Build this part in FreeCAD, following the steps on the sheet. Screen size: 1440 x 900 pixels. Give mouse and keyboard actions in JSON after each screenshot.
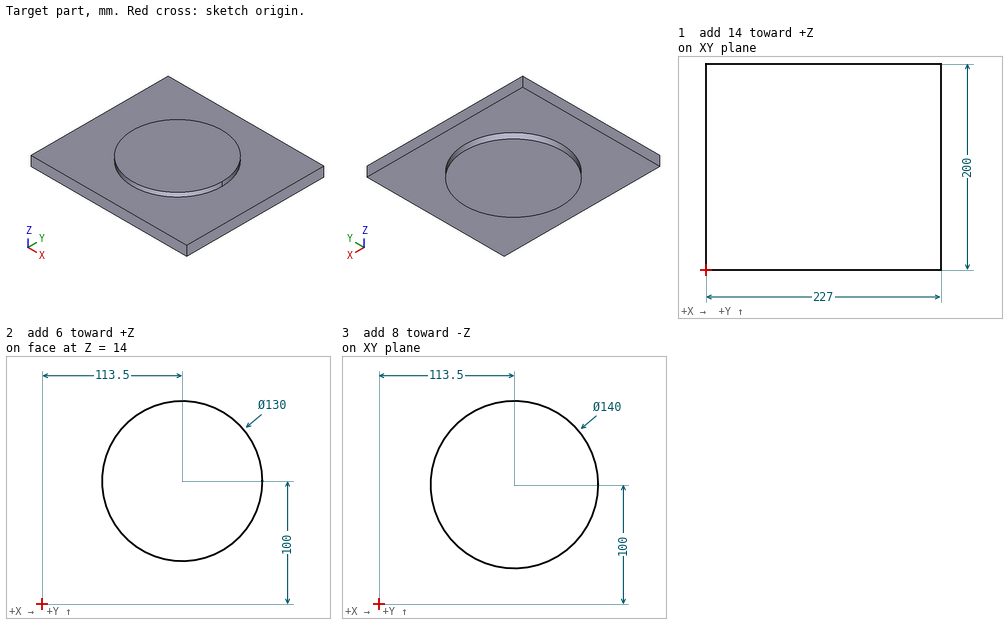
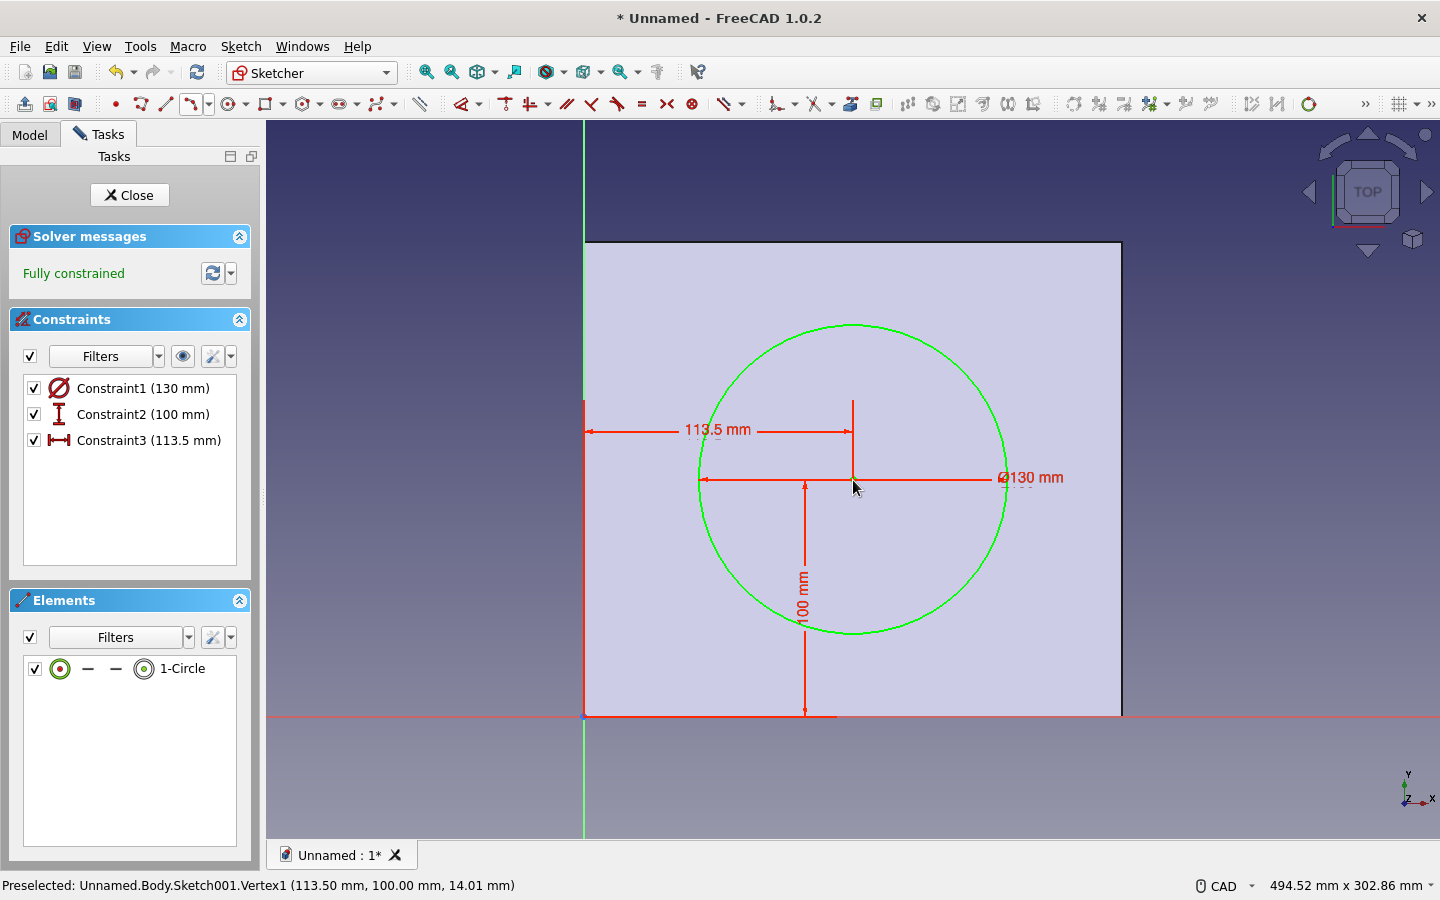
{"action": "left_click", "coordinate": [130, 195]}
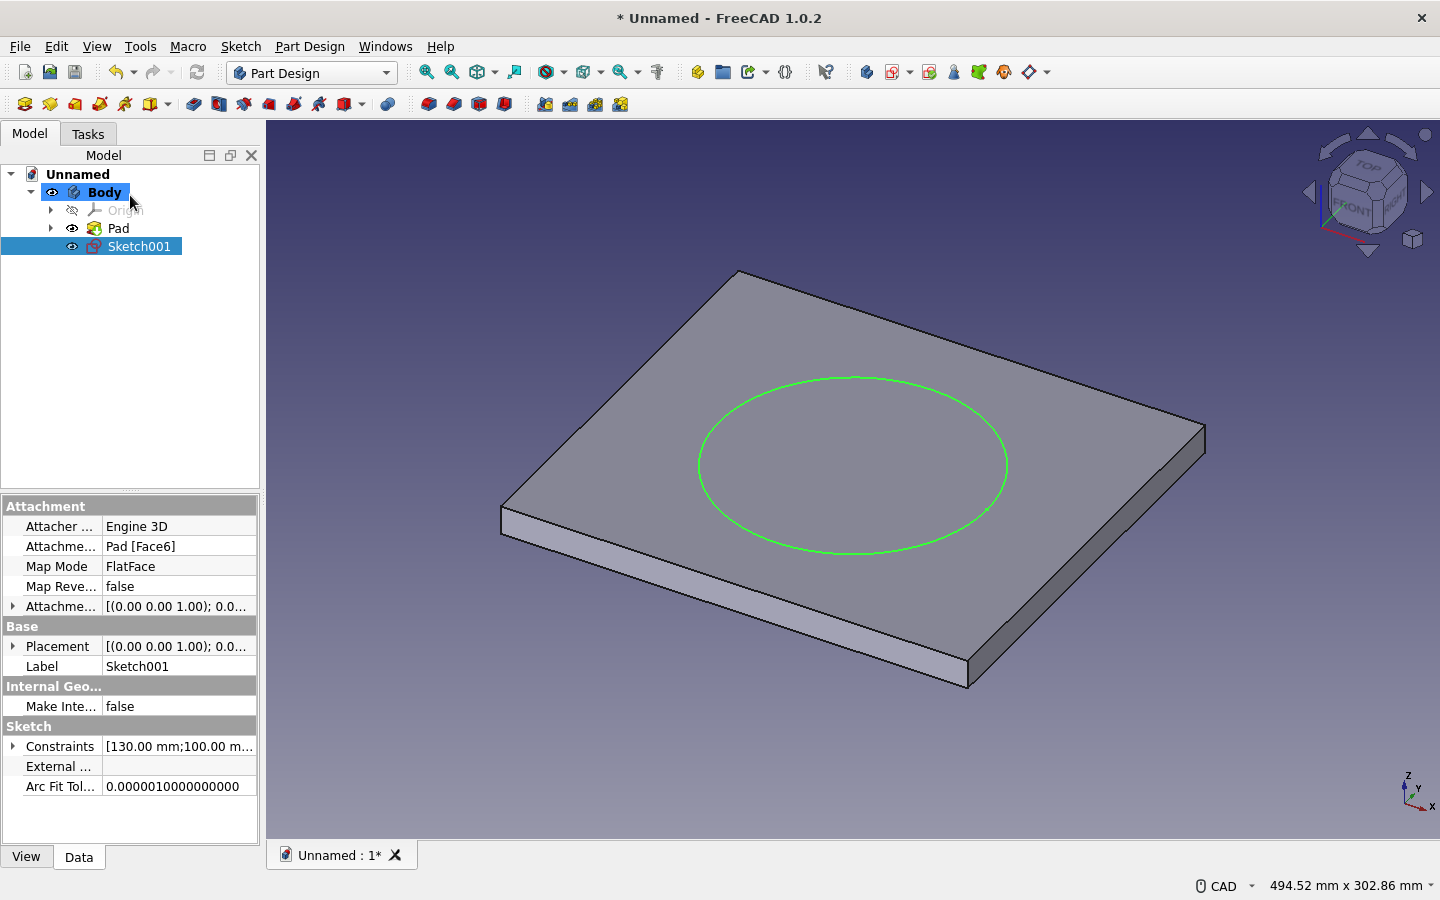
{"action": "left_click", "coordinate": [25, 104]}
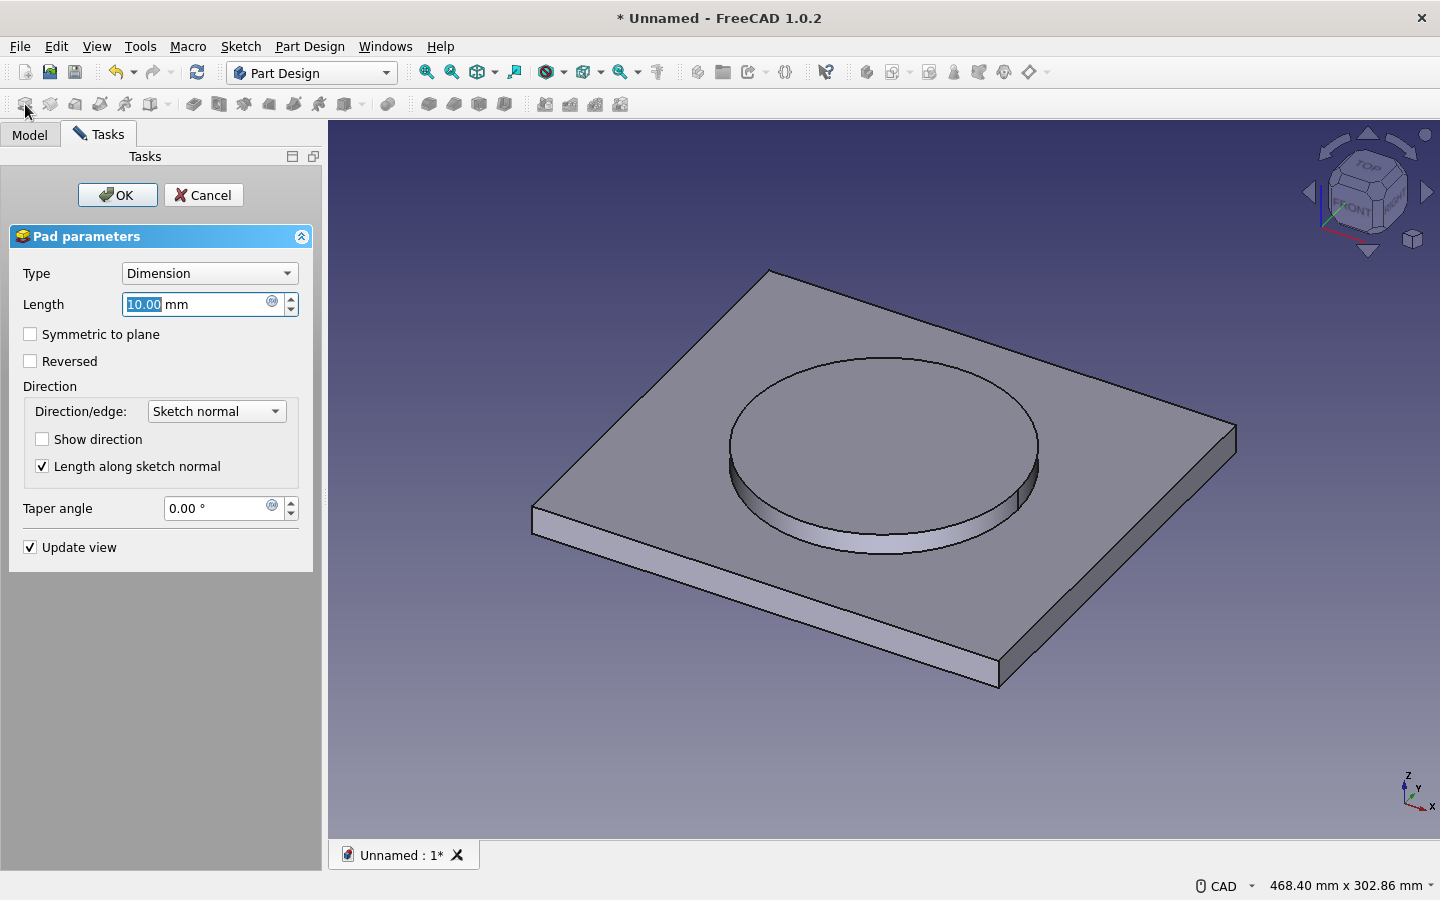
{"action": "type", "text": "6"}
{"action": "key", "text": "Tab"}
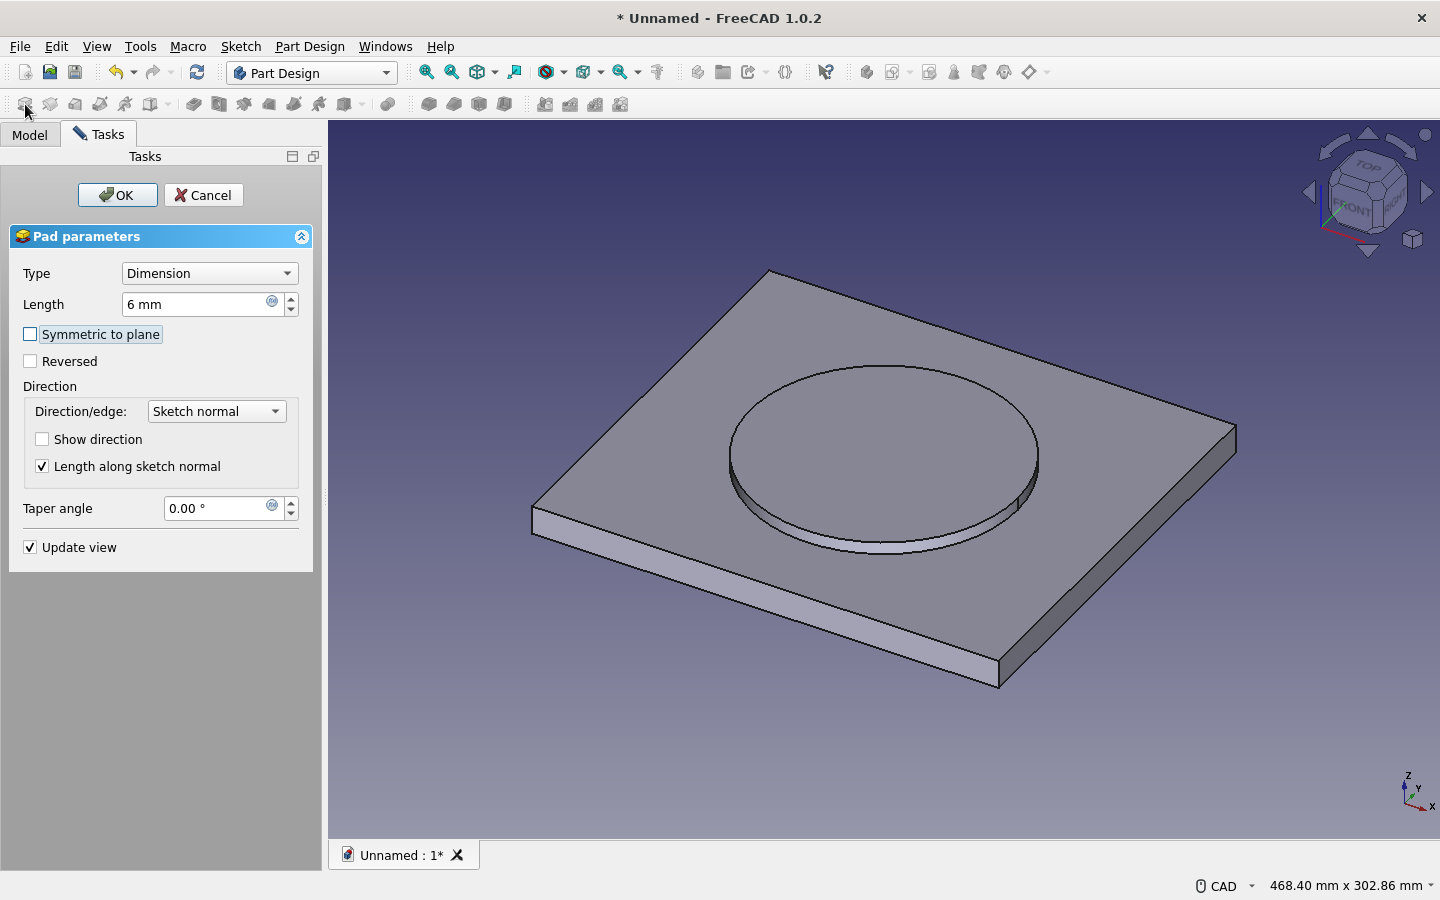
{"action": "left_click", "coordinate": [118, 195]}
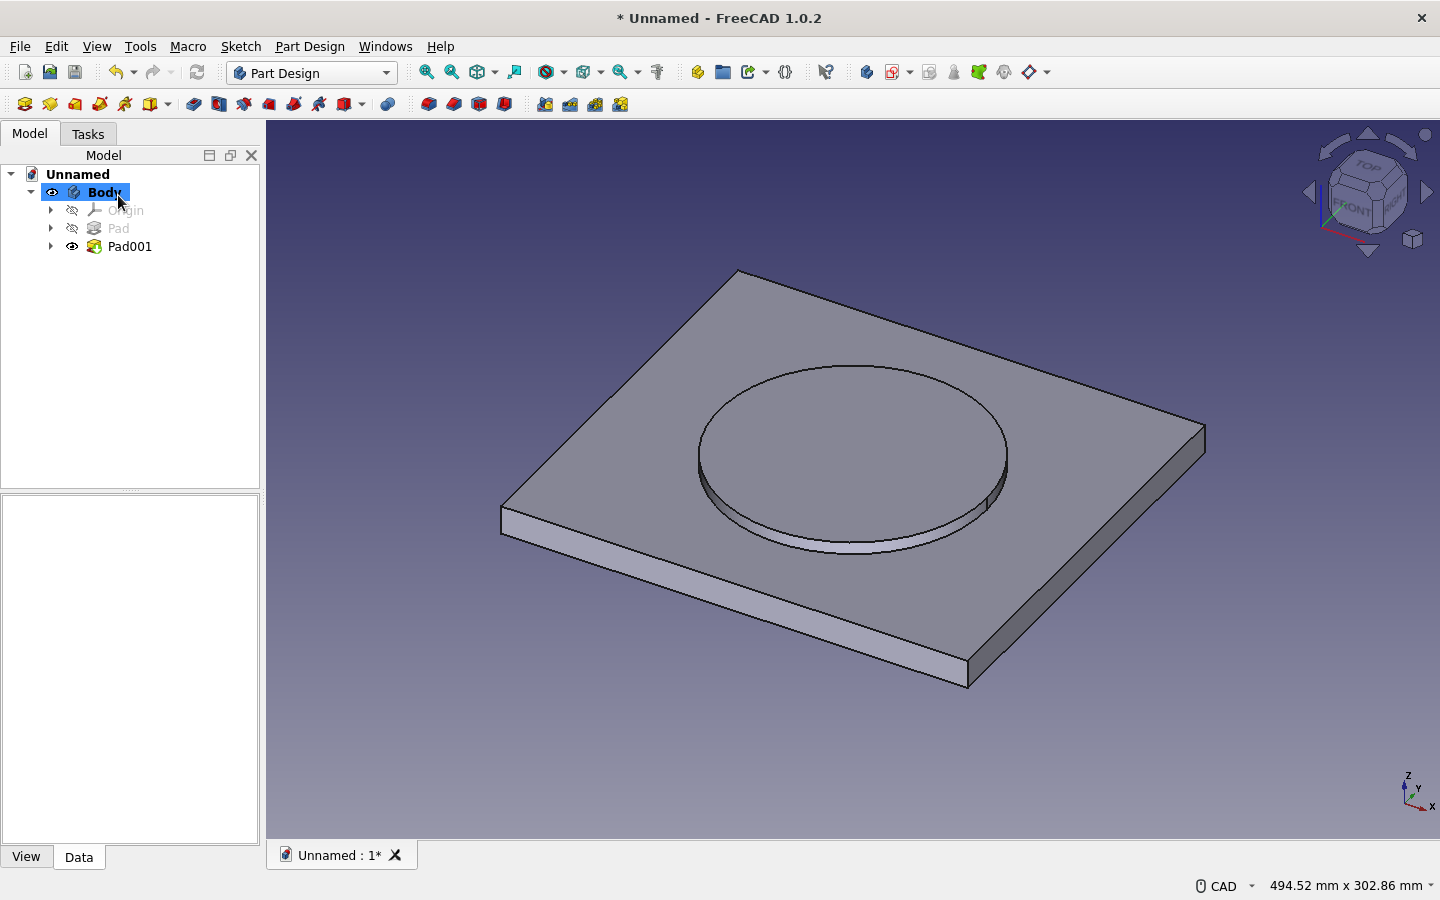
{"action": "left_click", "coordinate": [892, 72]}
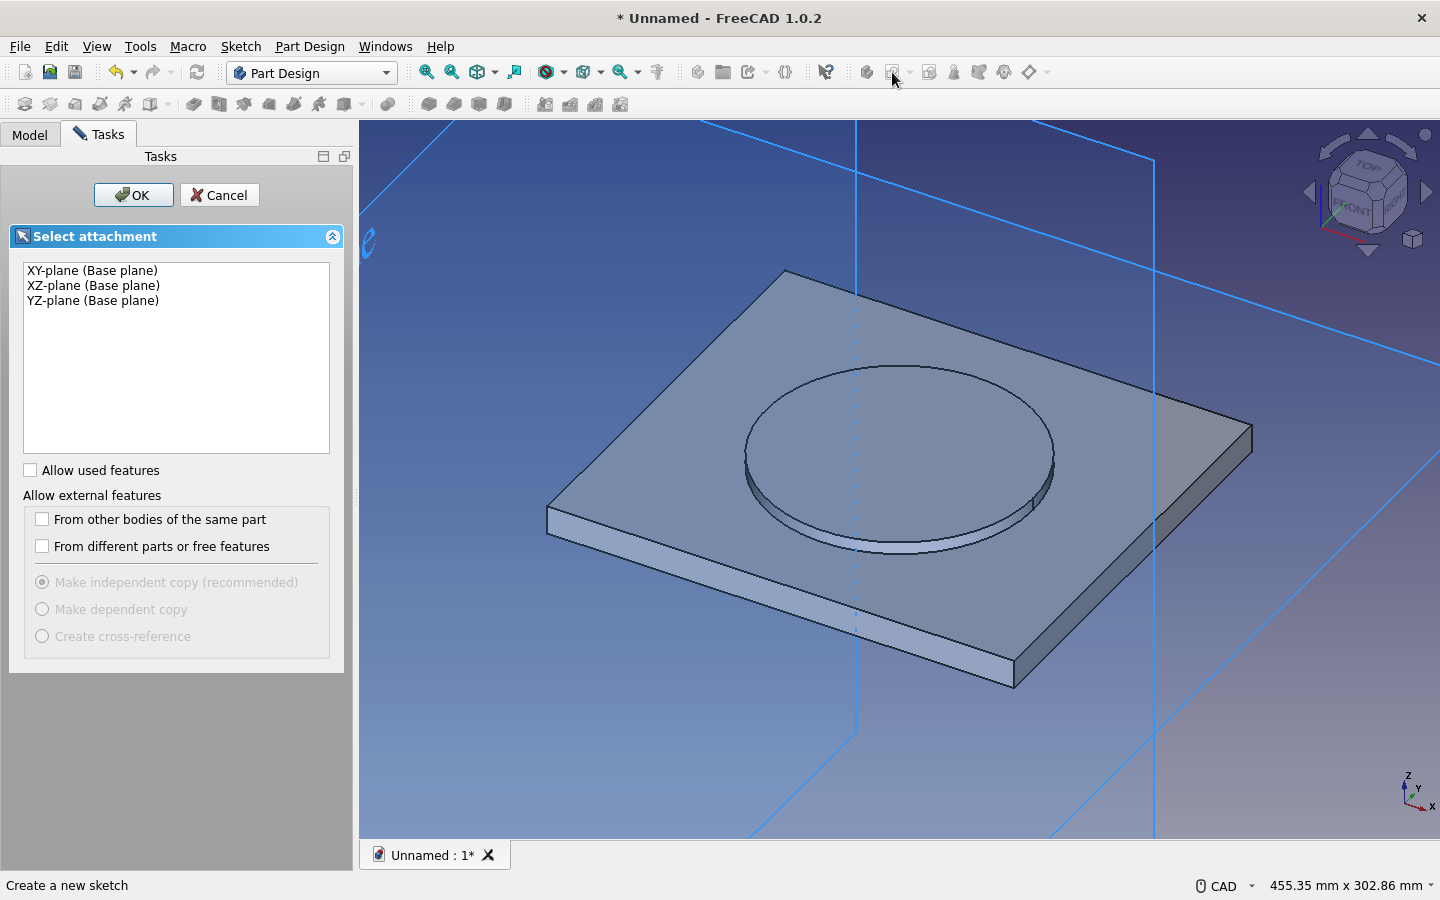
{"action": "left_click", "coordinate": [84, 270]}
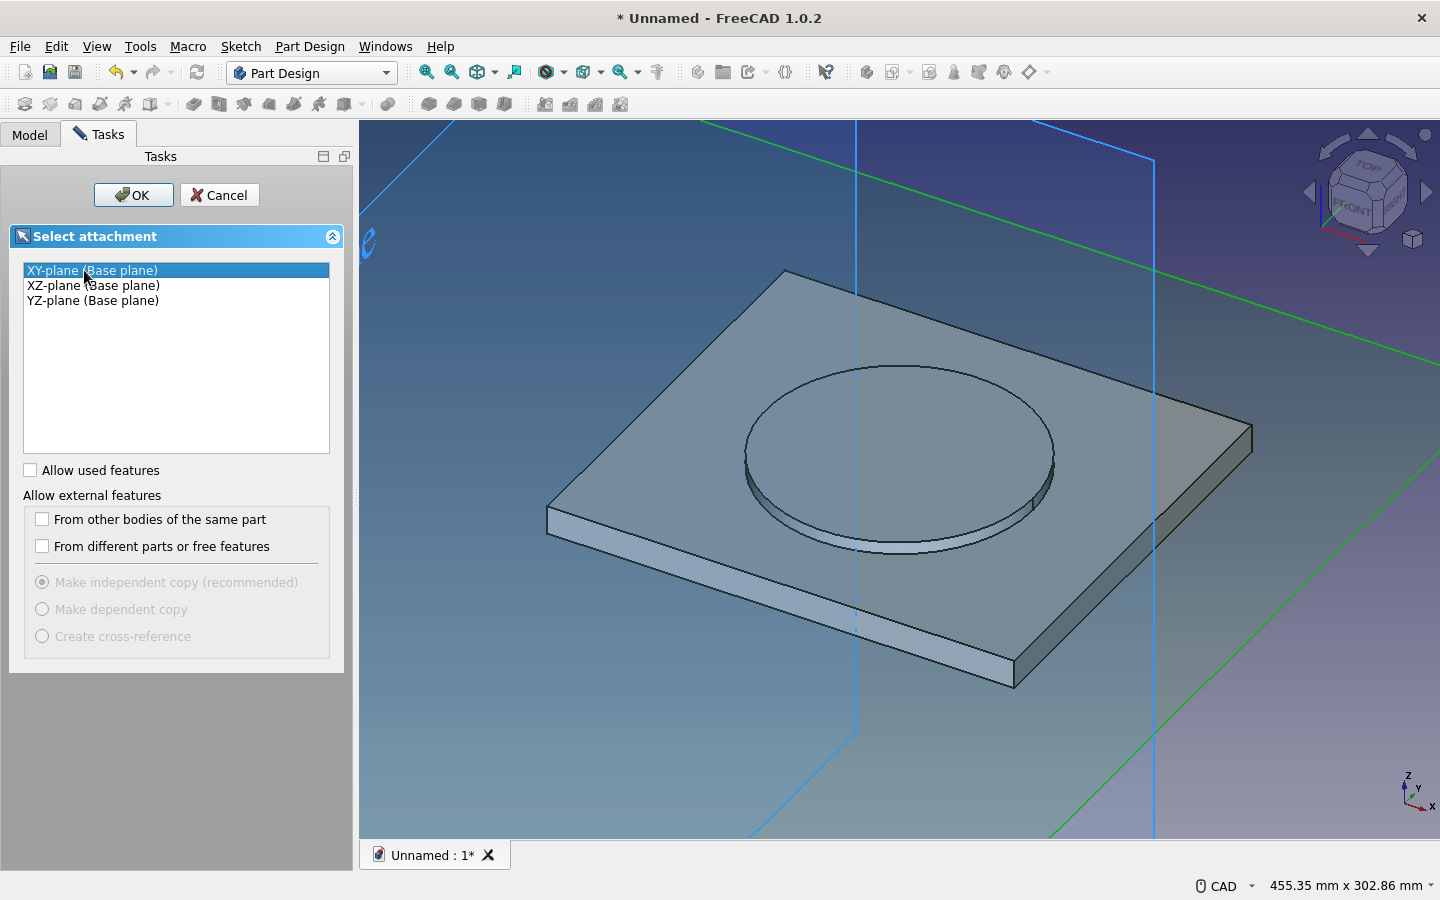
{"action": "left_click", "coordinate": [134, 195]}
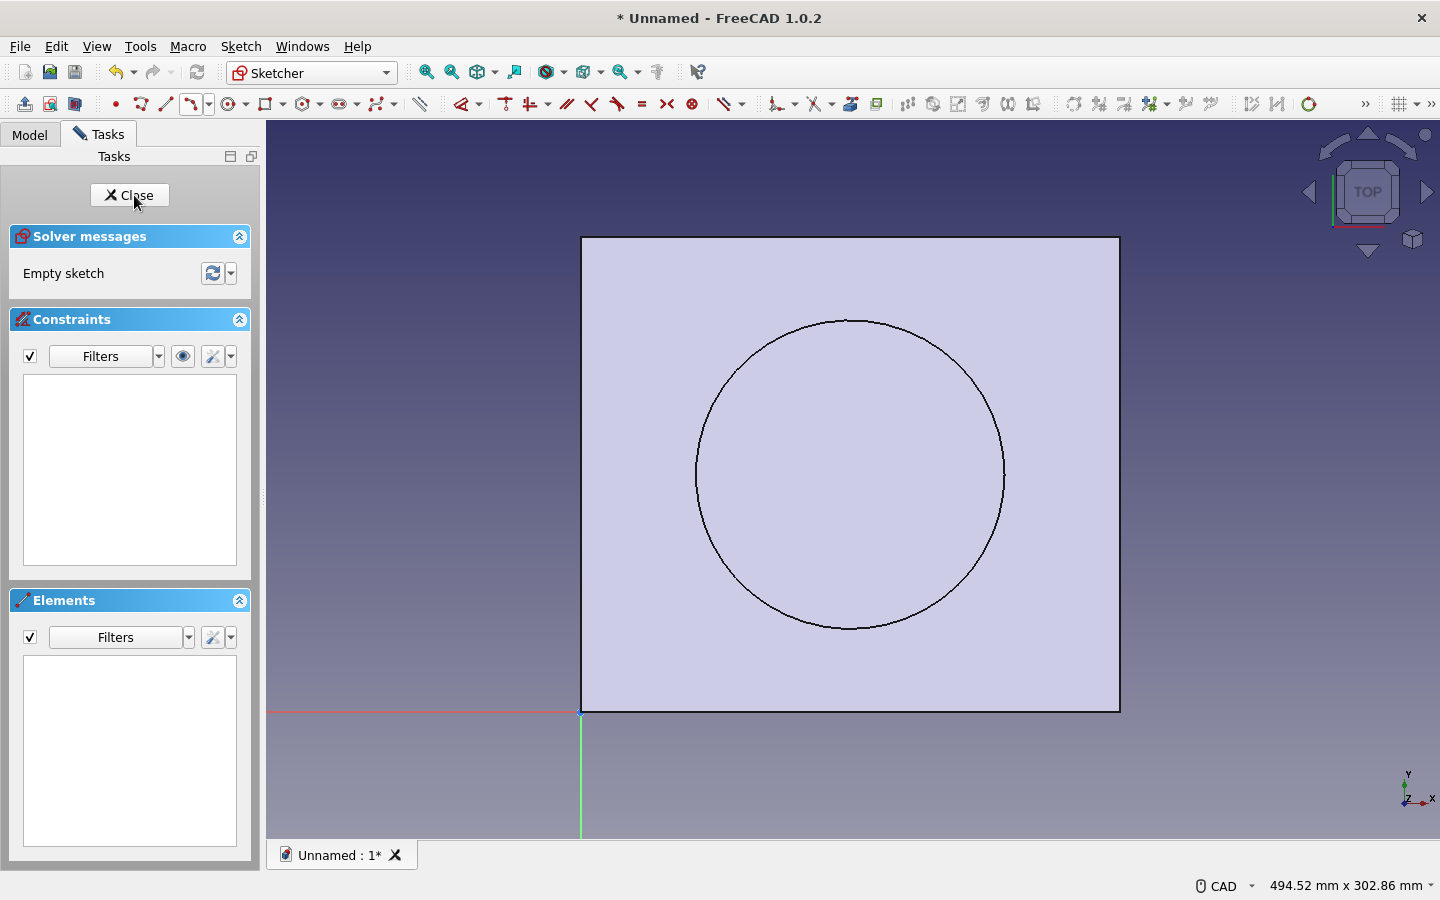
{"action": "key", "text": "q s"}